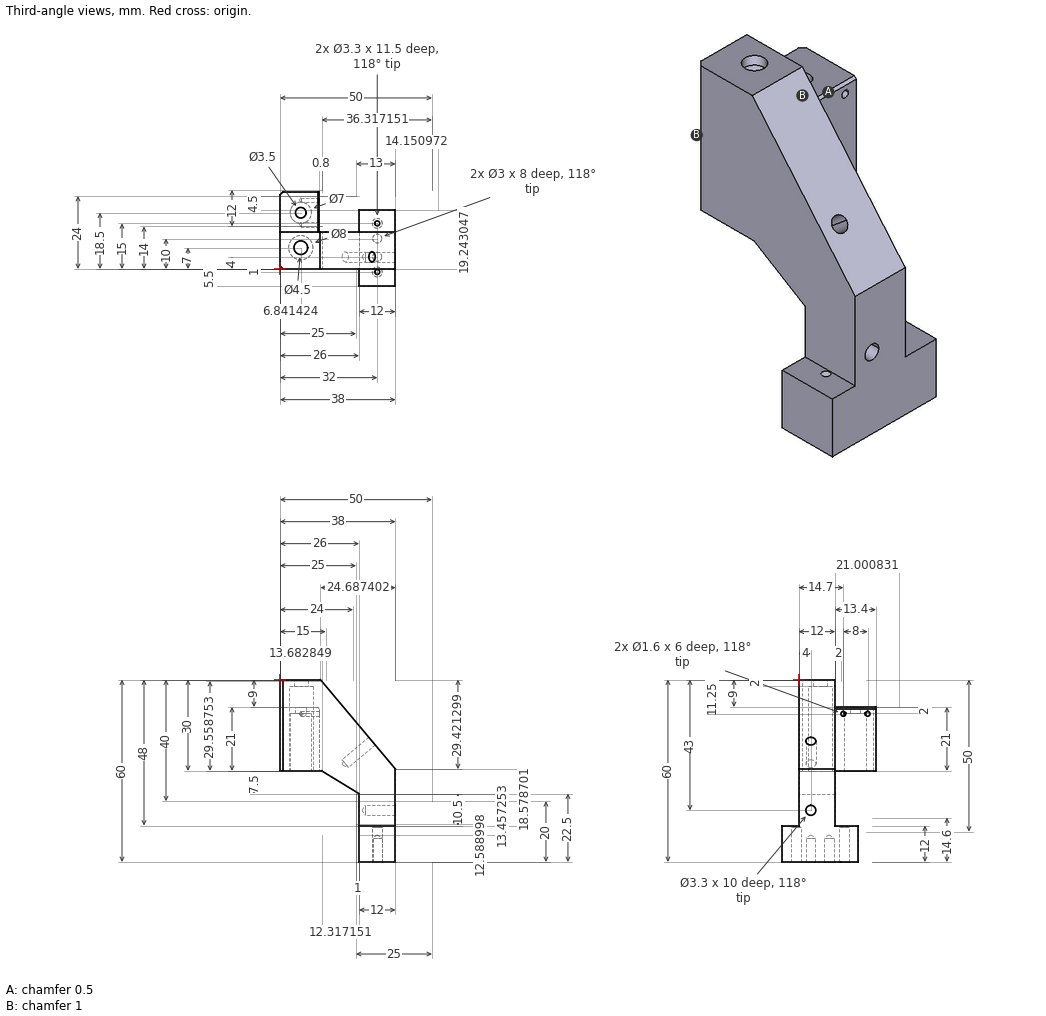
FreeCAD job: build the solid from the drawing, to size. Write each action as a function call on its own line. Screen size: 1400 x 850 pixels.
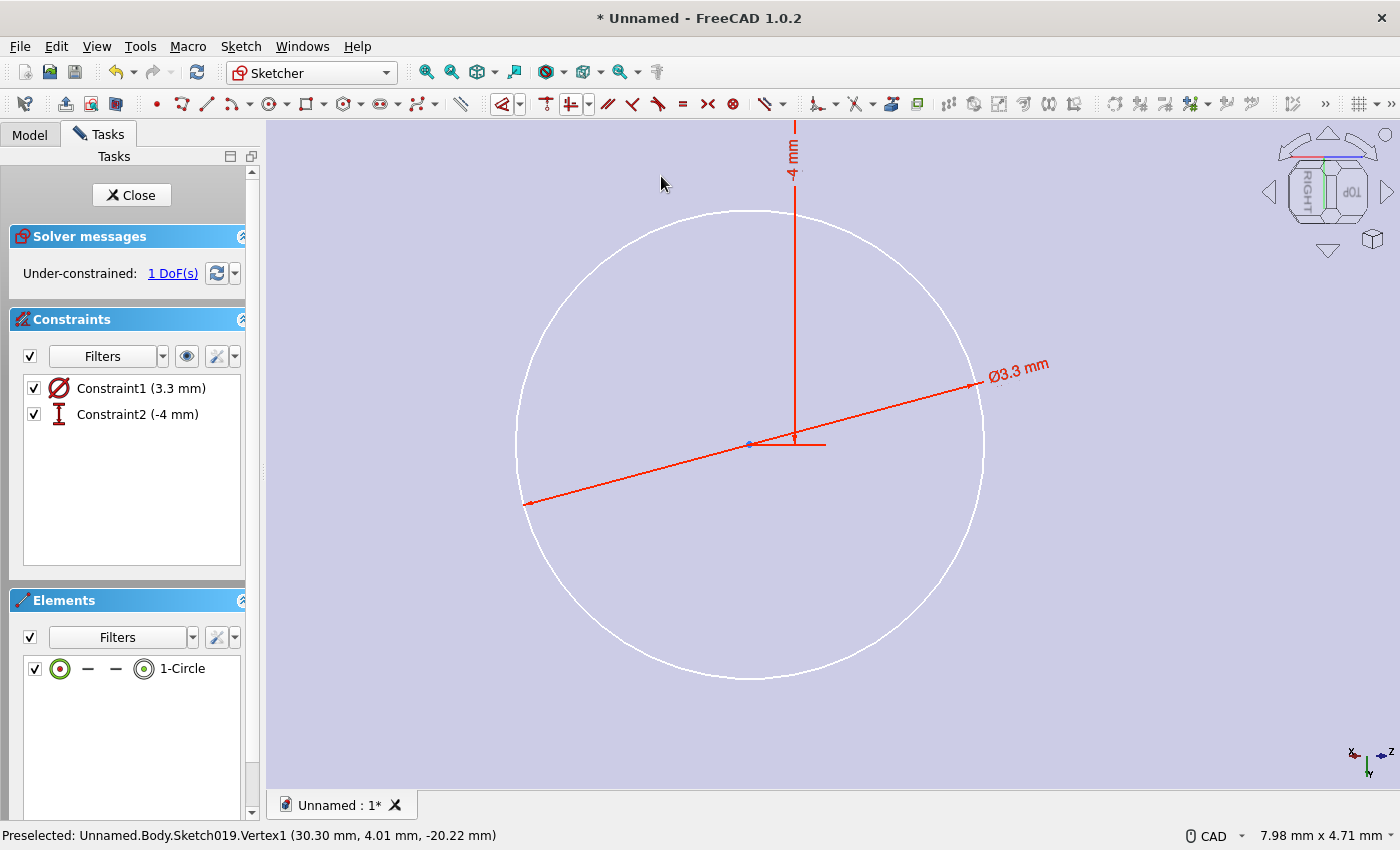
click(750, 445)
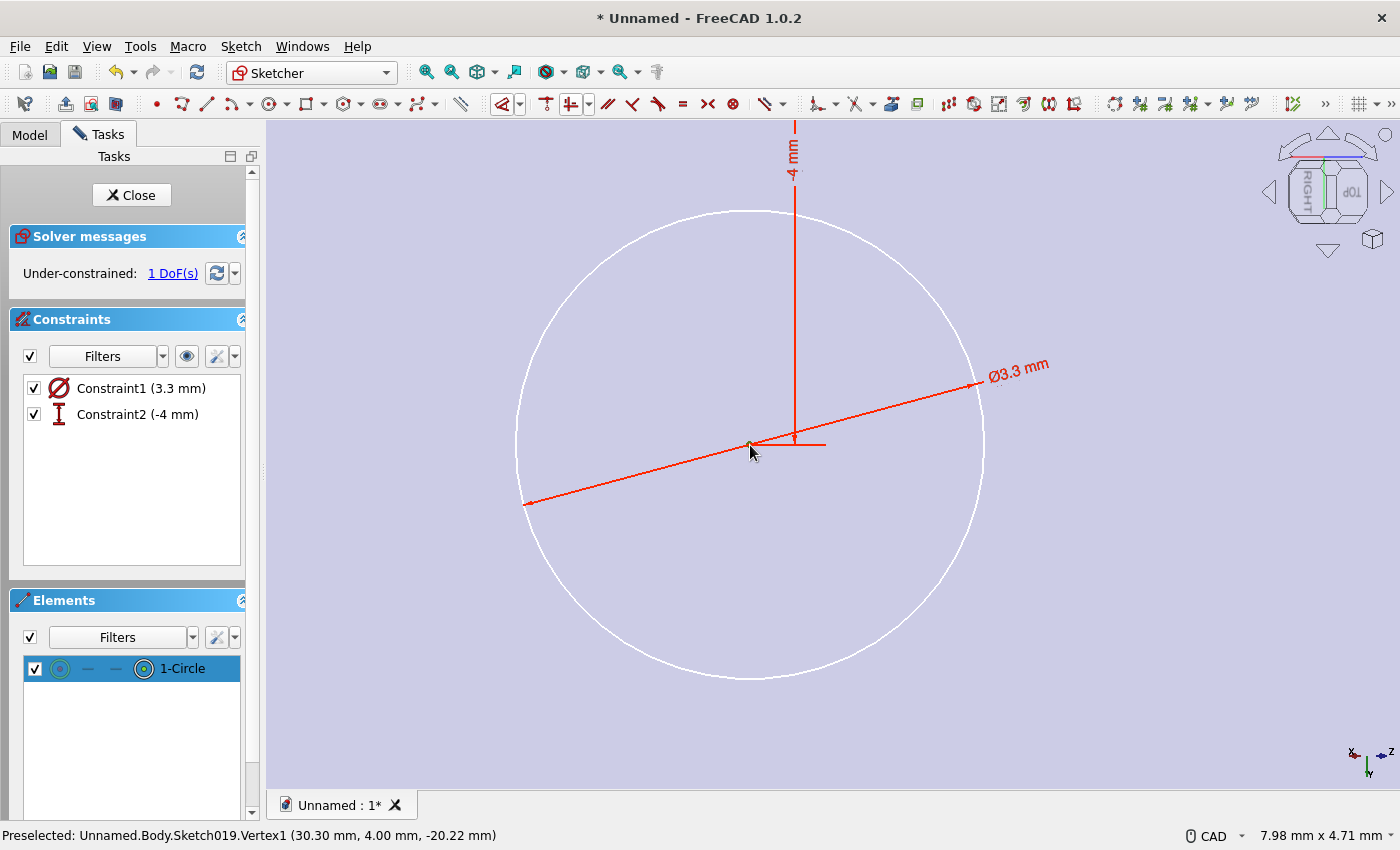
click(520, 104)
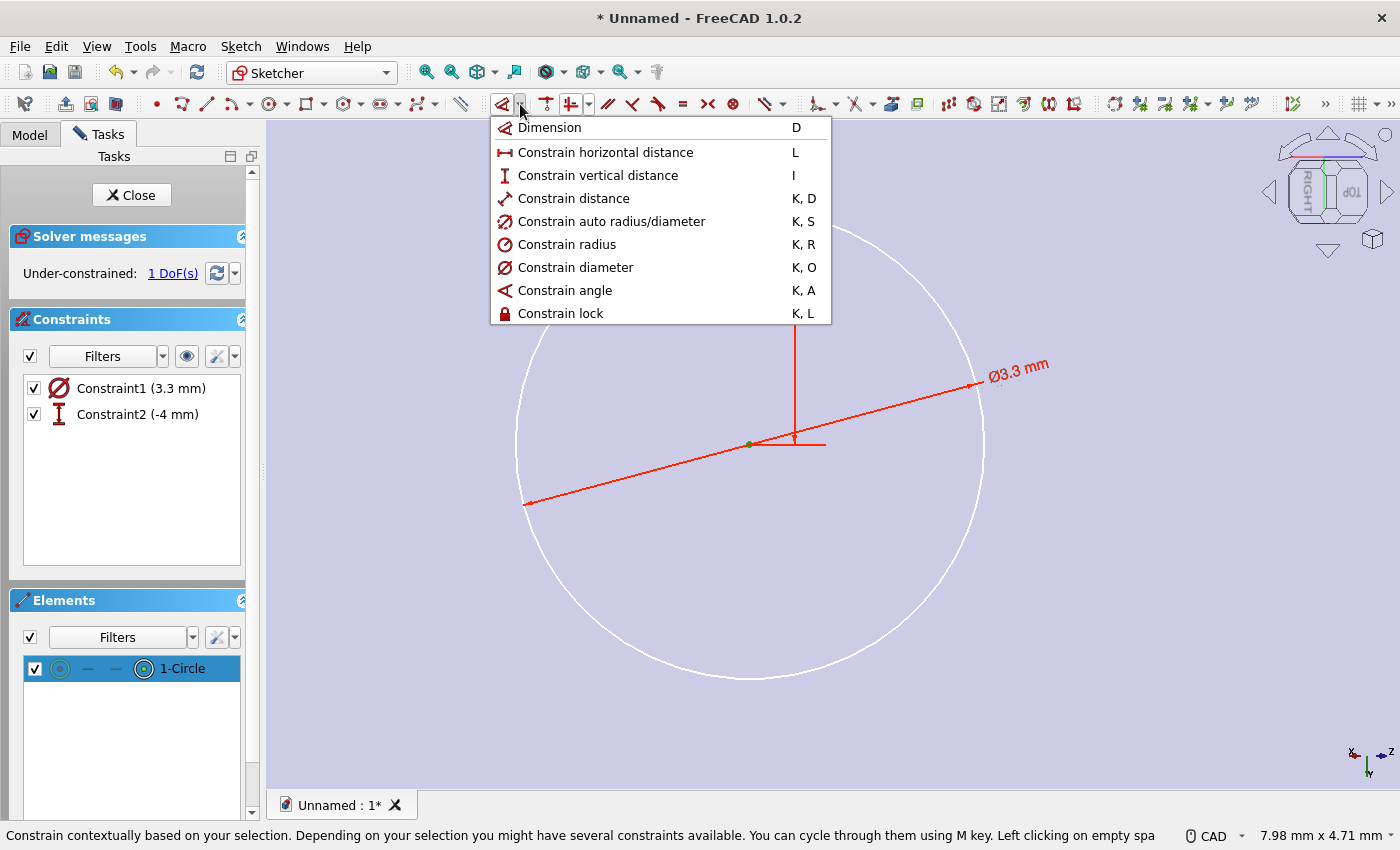
click(661, 152)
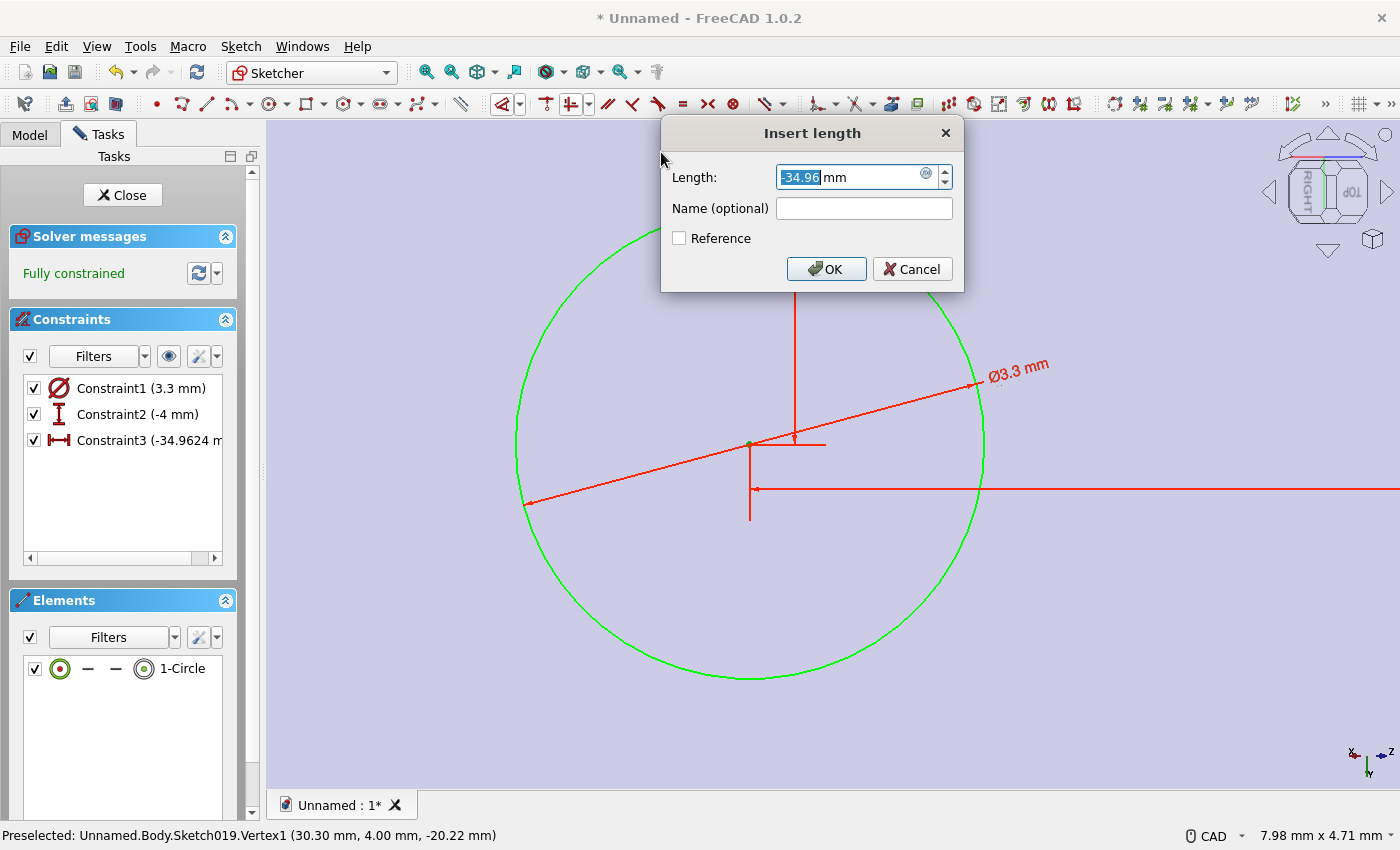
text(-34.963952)
key(Return)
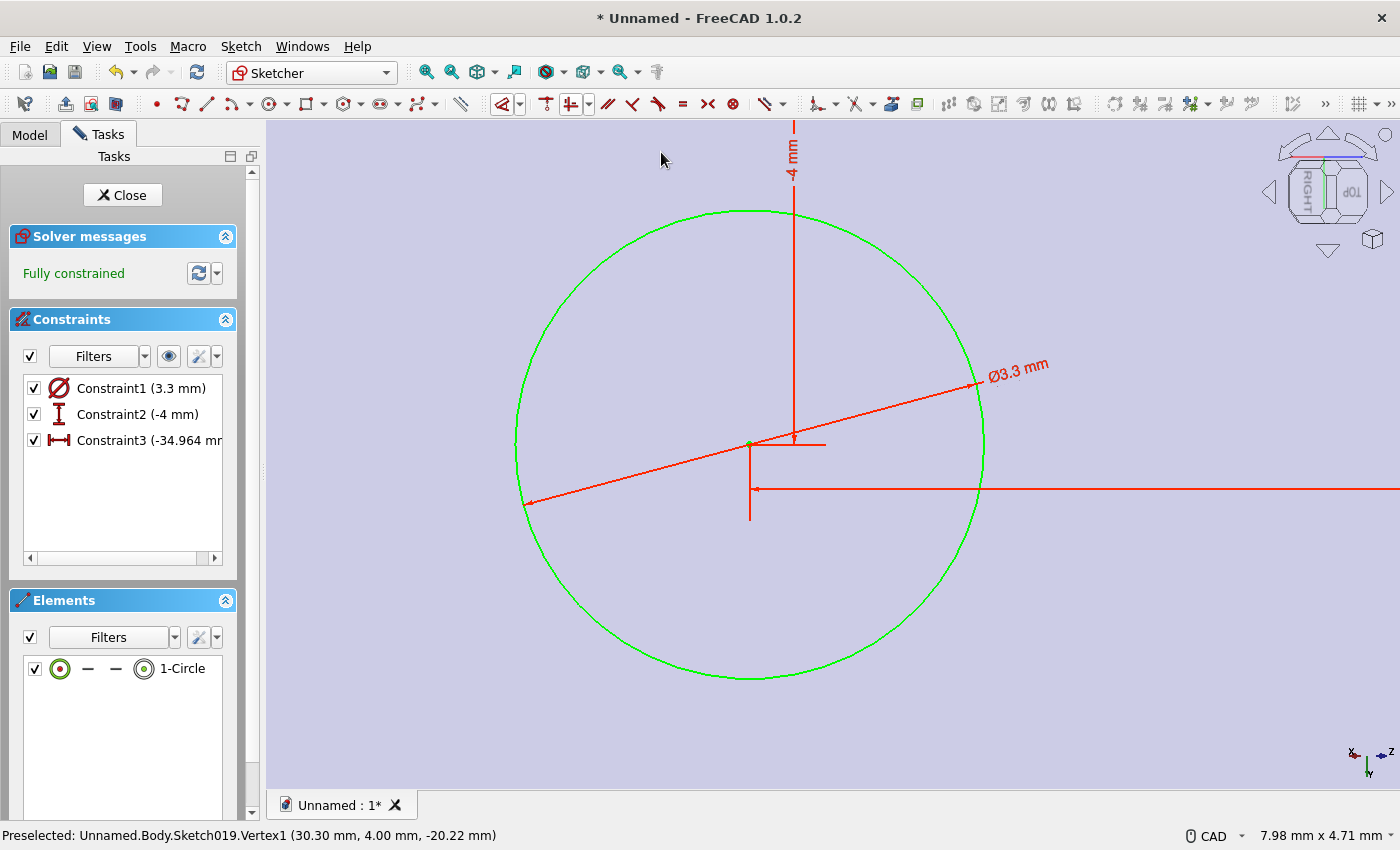
click(123, 195)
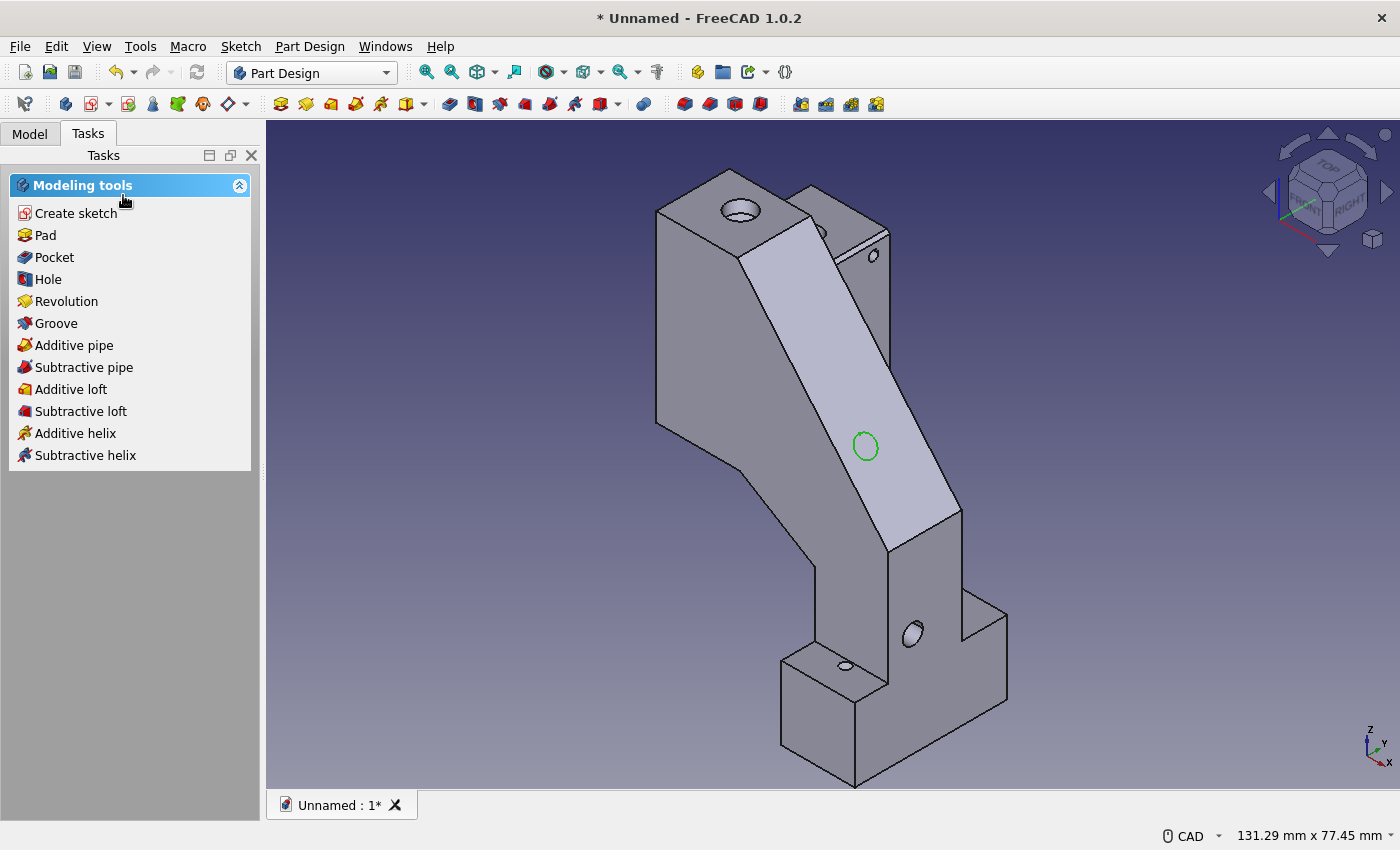
click(475, 104)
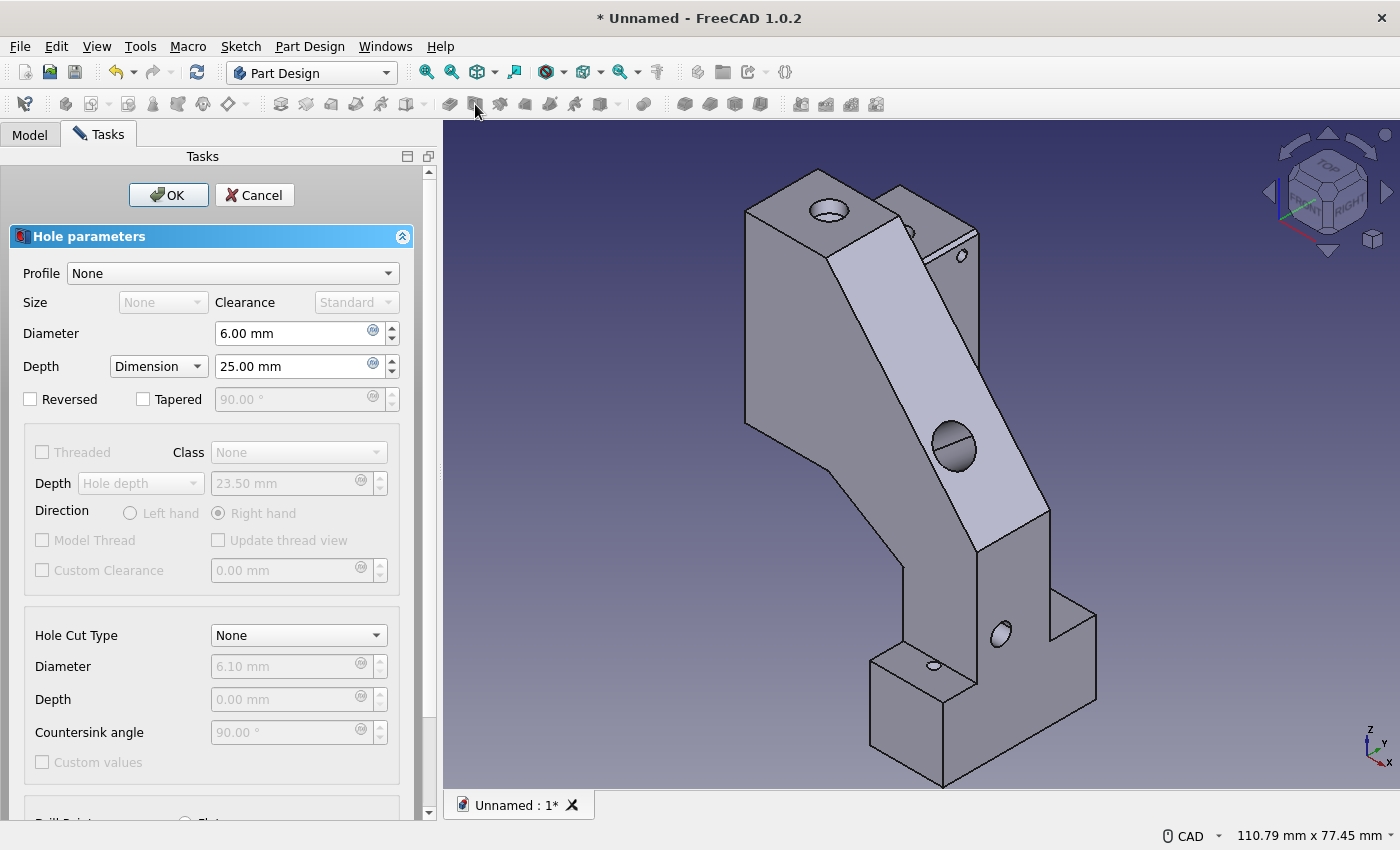
triple_click(300, 334)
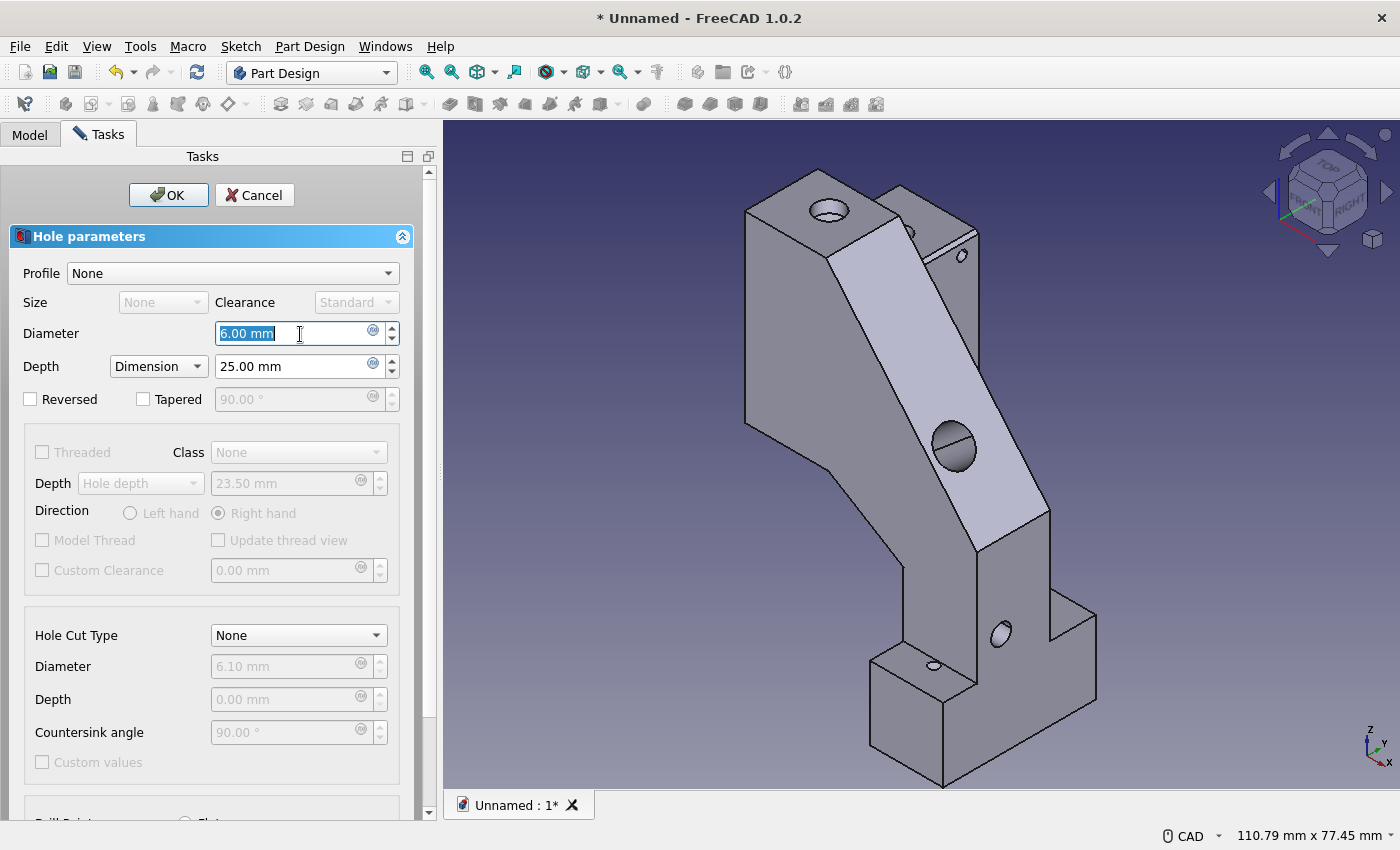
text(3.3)
key(Tab)